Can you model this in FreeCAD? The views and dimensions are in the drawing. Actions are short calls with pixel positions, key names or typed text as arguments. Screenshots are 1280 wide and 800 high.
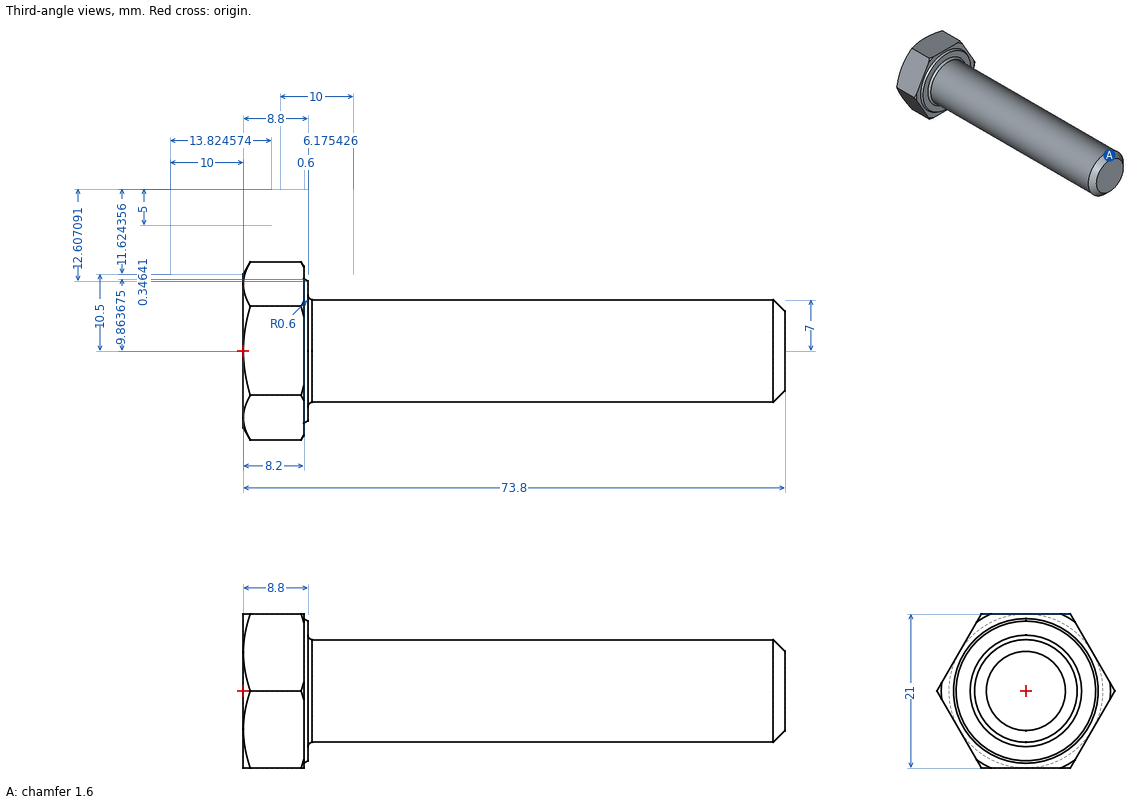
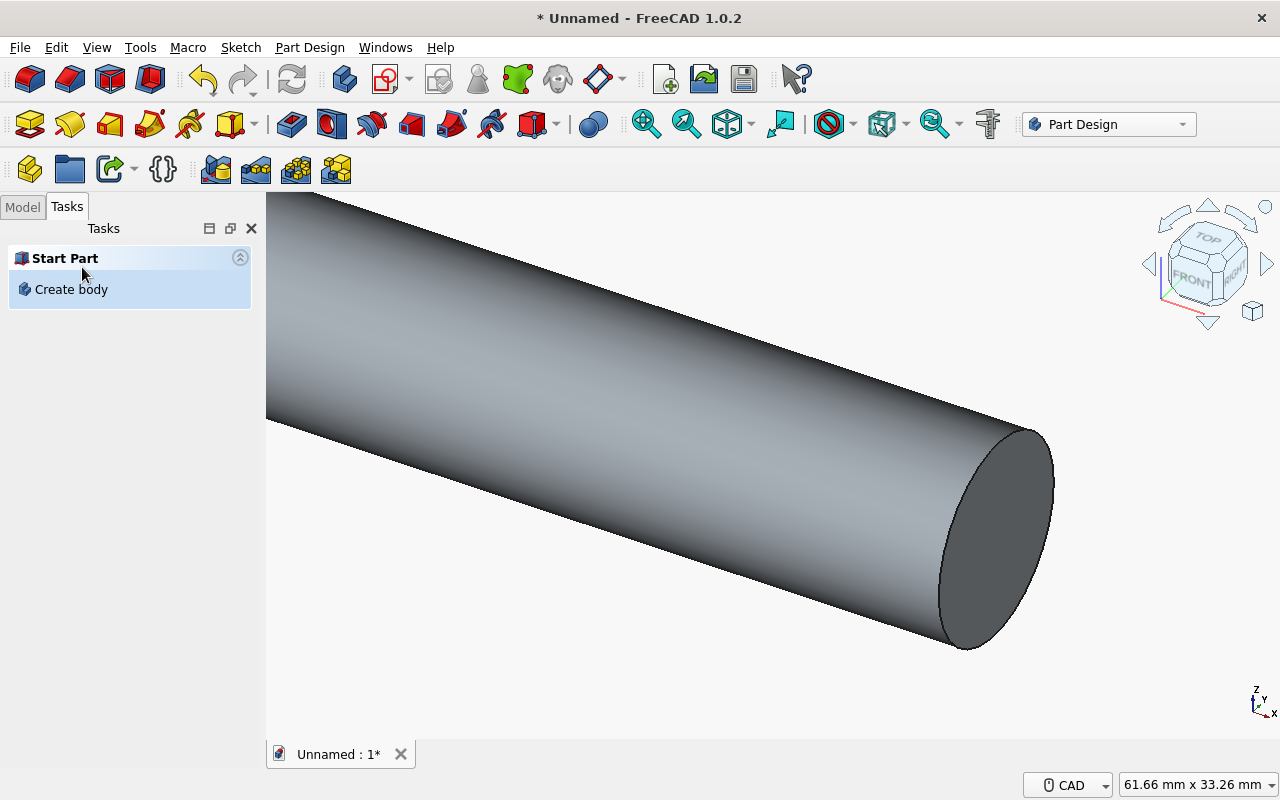
click(648, 124)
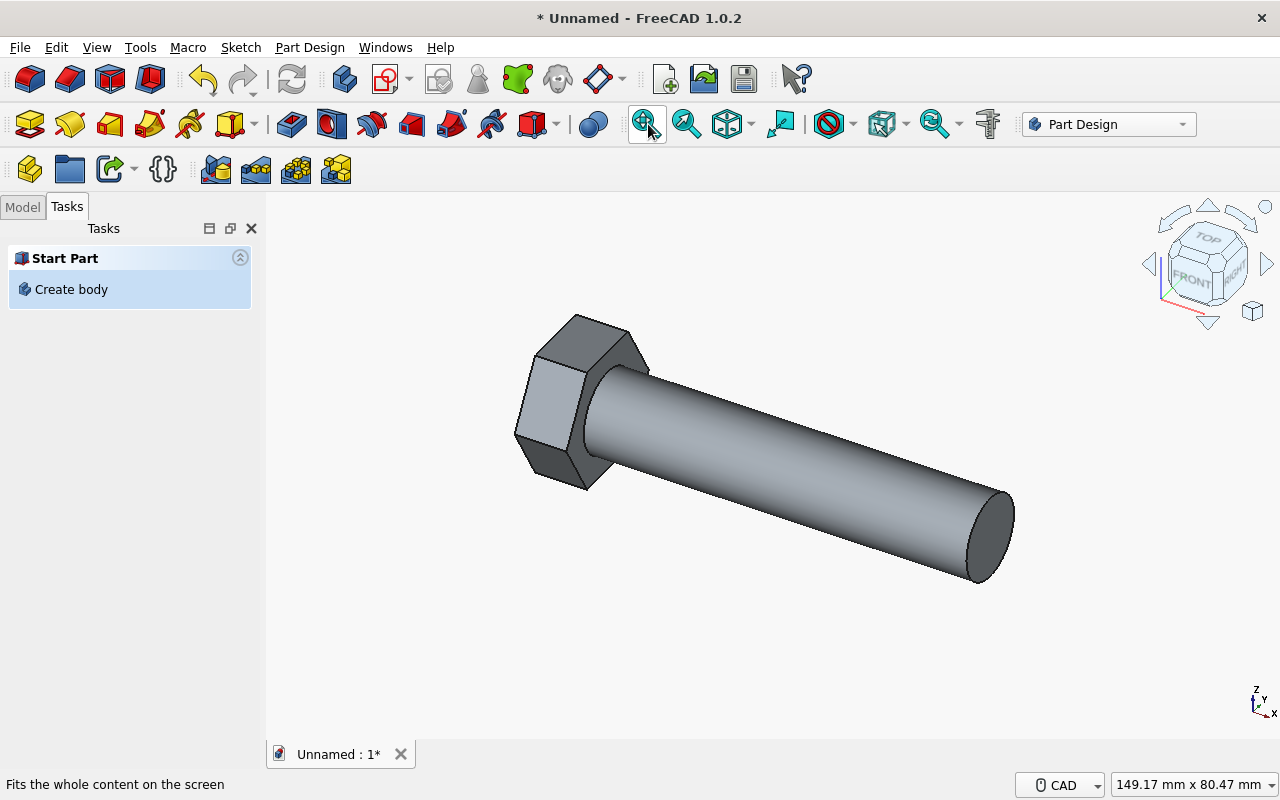
click(386, 80)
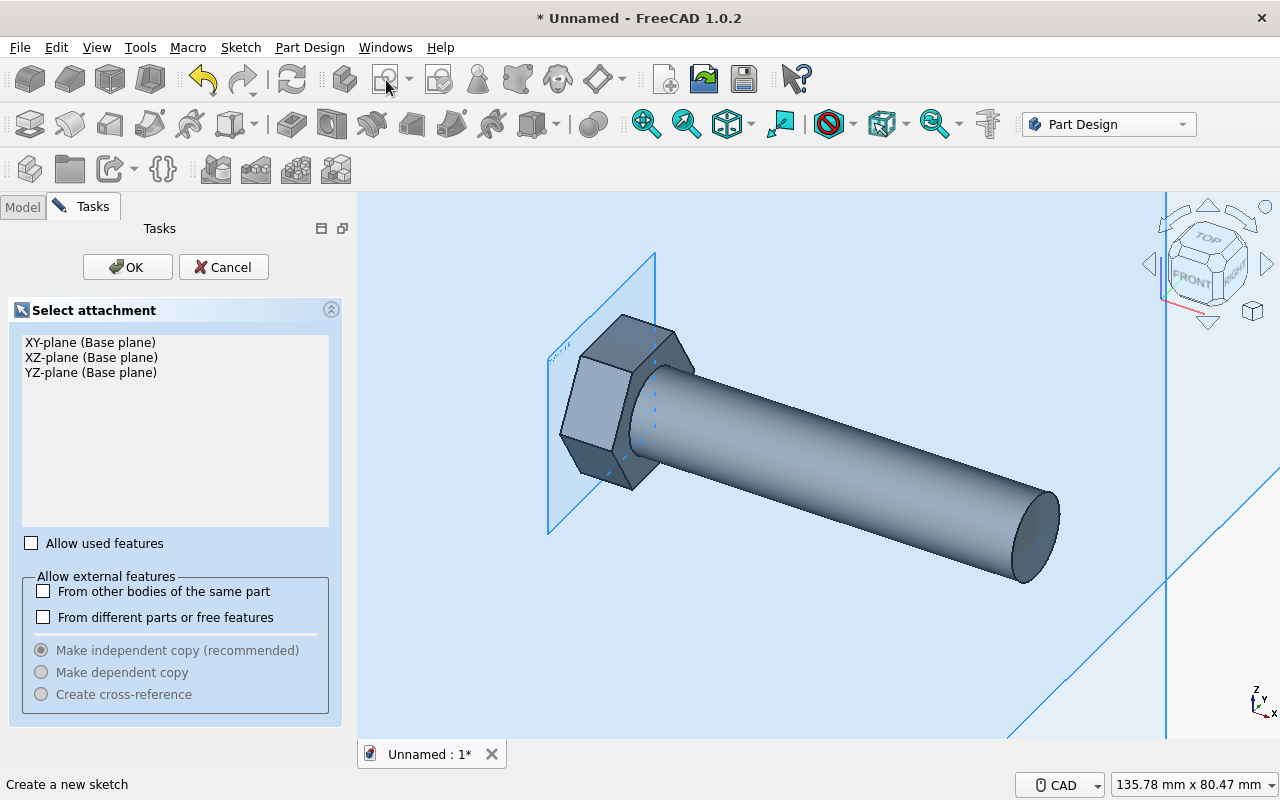
click(82, 342)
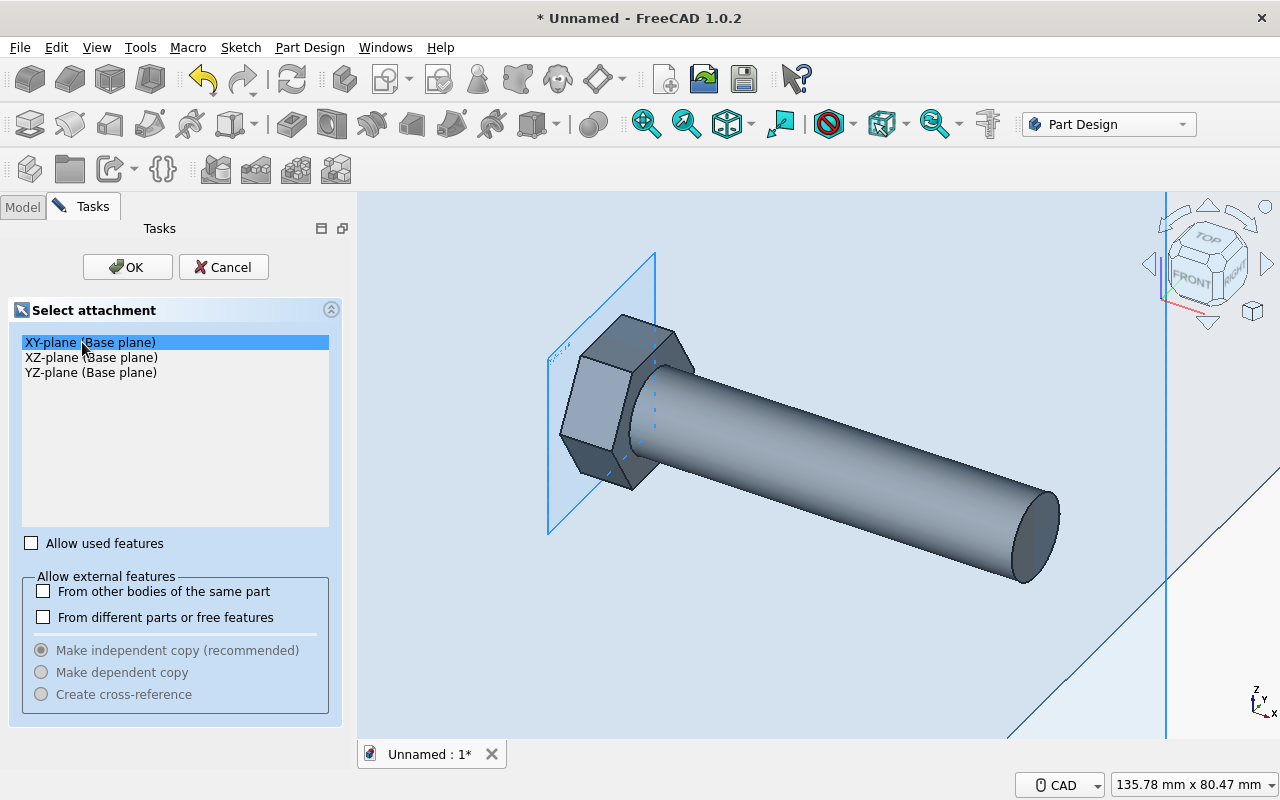
click(128, 267)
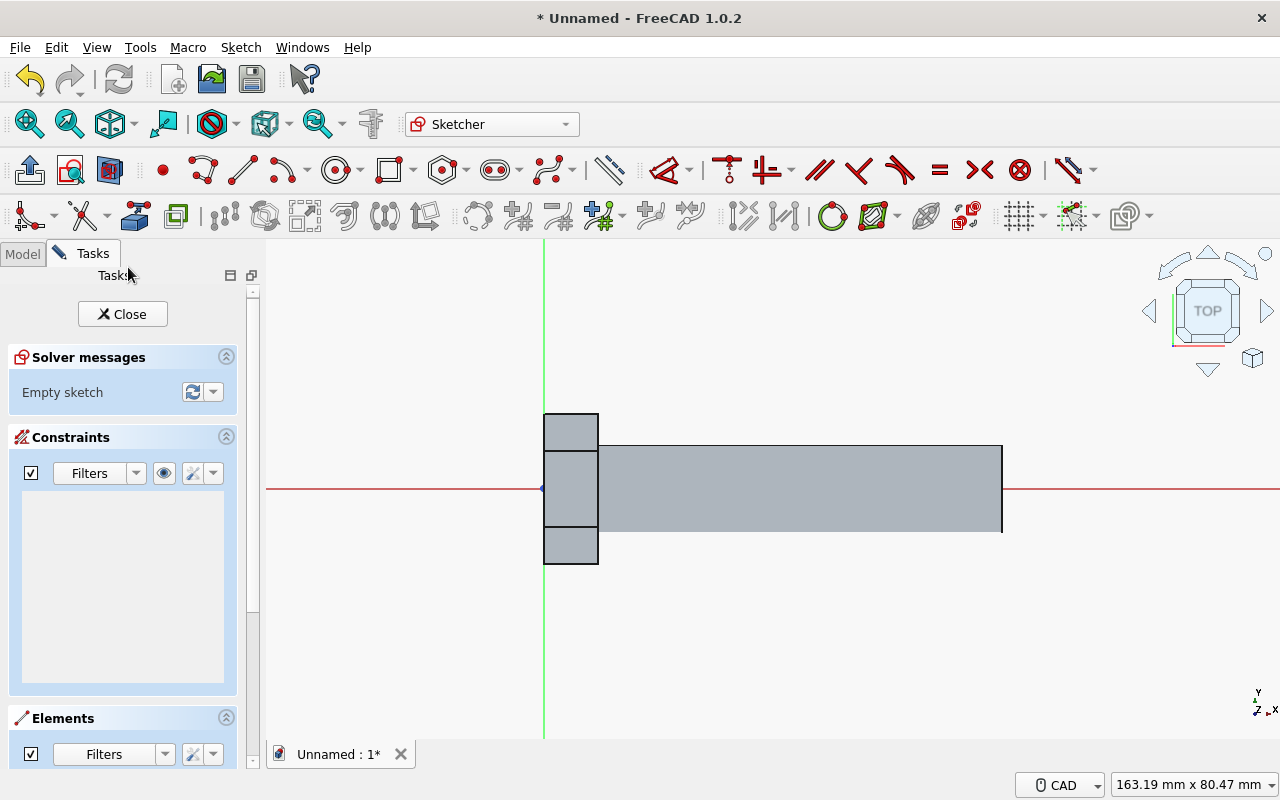
click(110, 170)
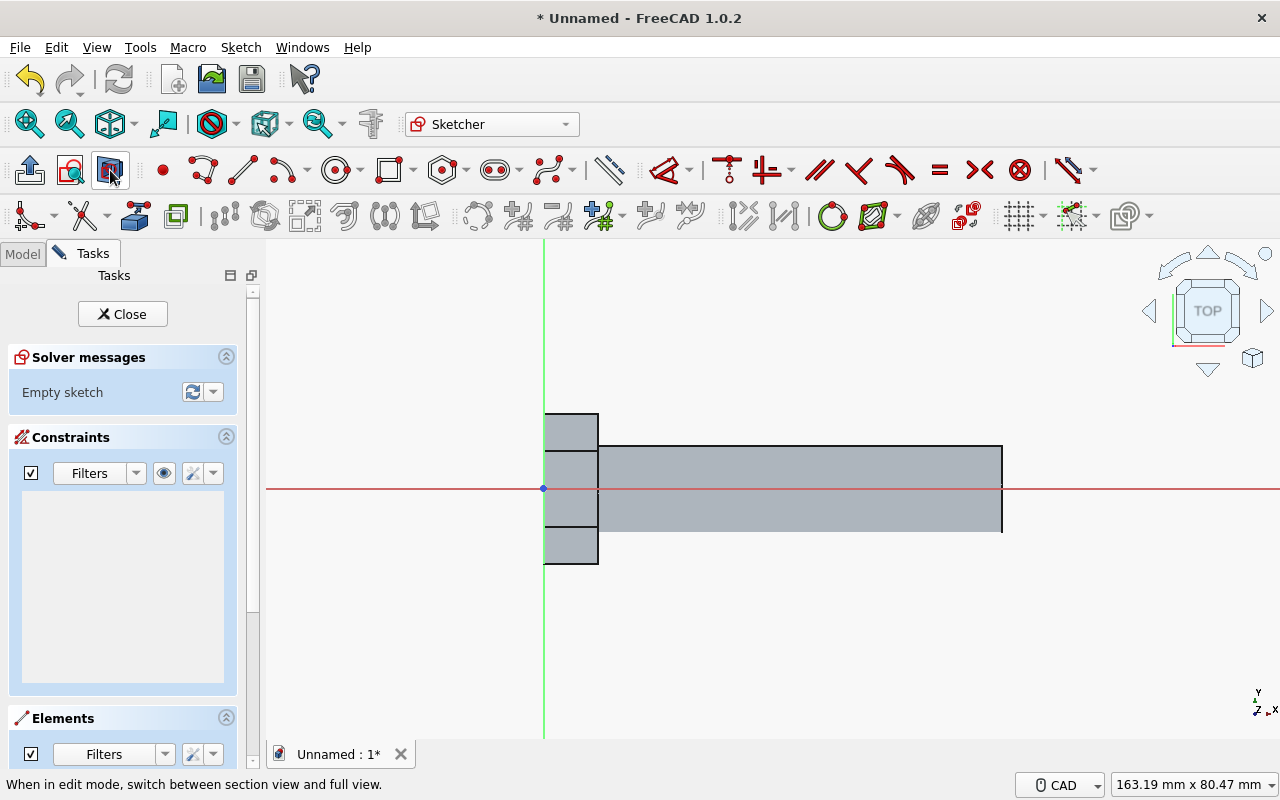
scroll(378, 364, up, 4)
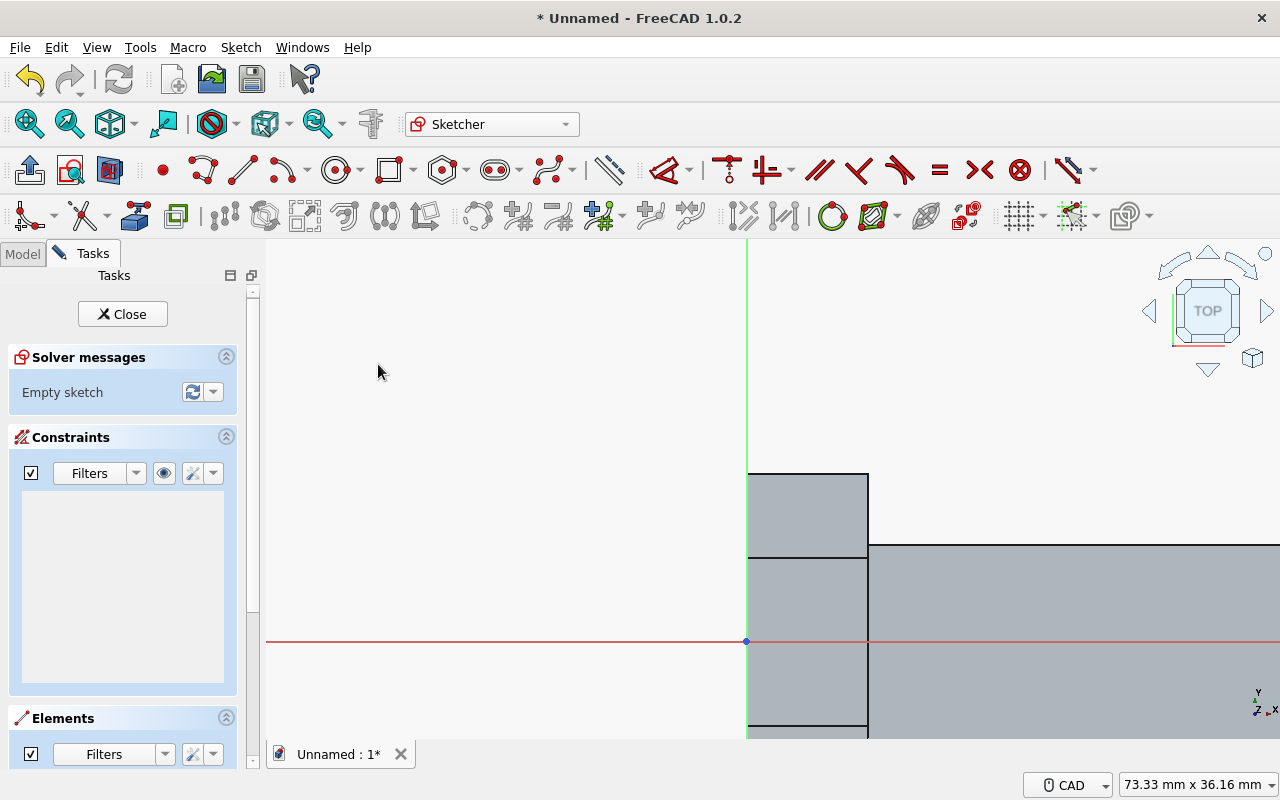
click(204, 170)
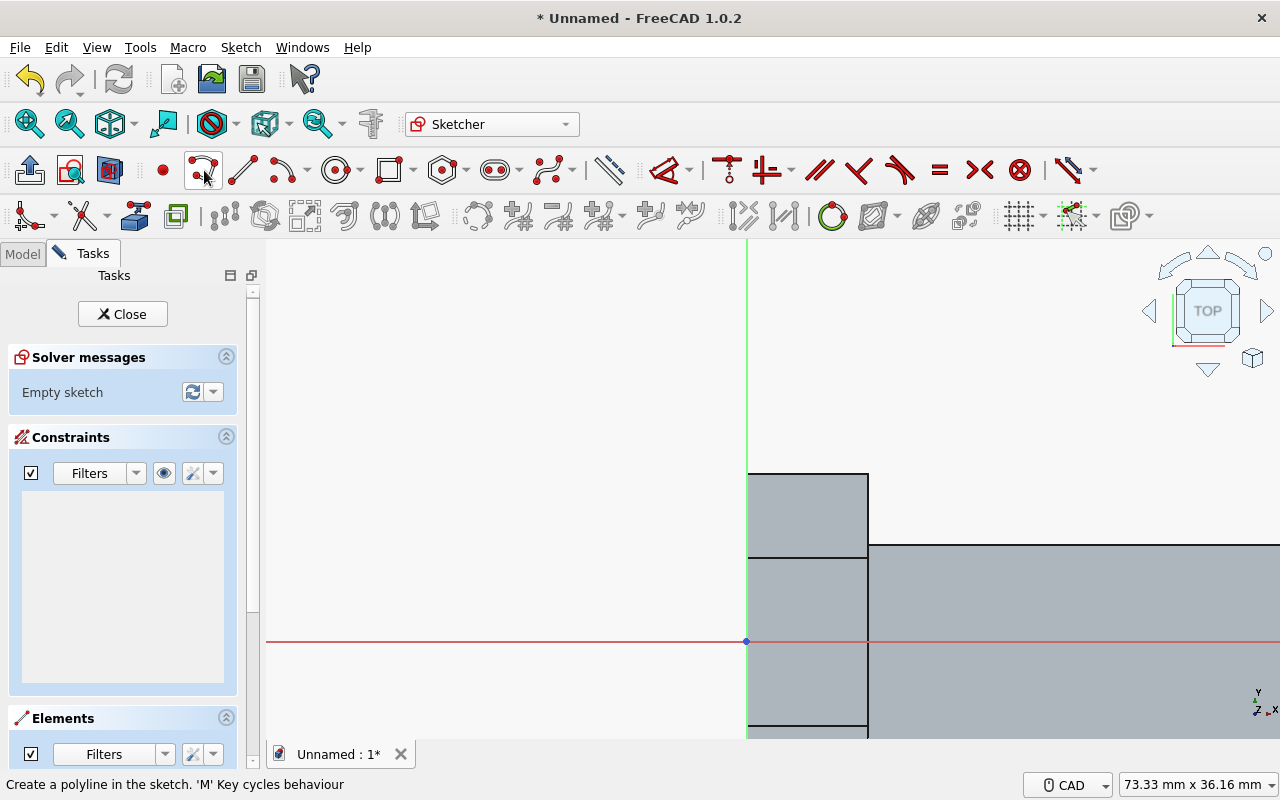
click(747, 497)
click(800, 405)
click(800, 336)
click(608, 336)
click(608, 497)
click(747, 498)
key(Escape)
key(Escape)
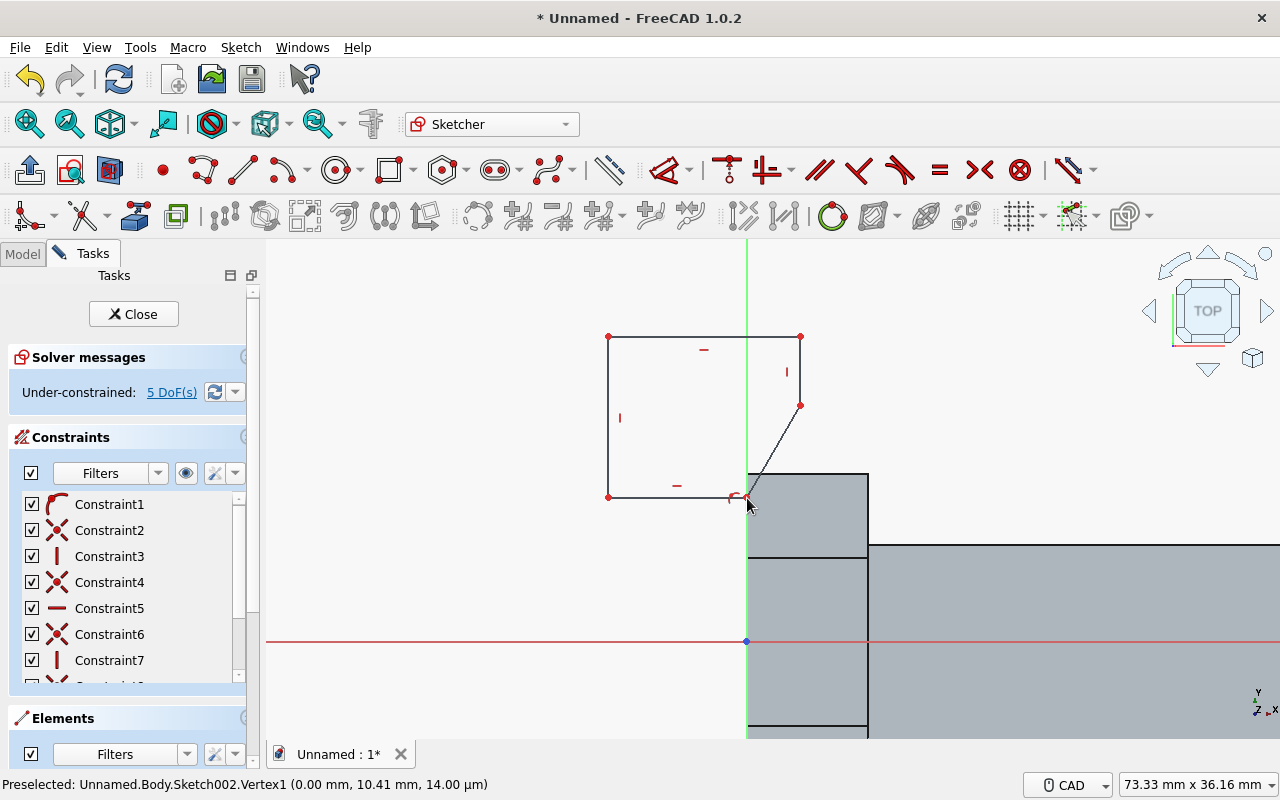
click(664, 170)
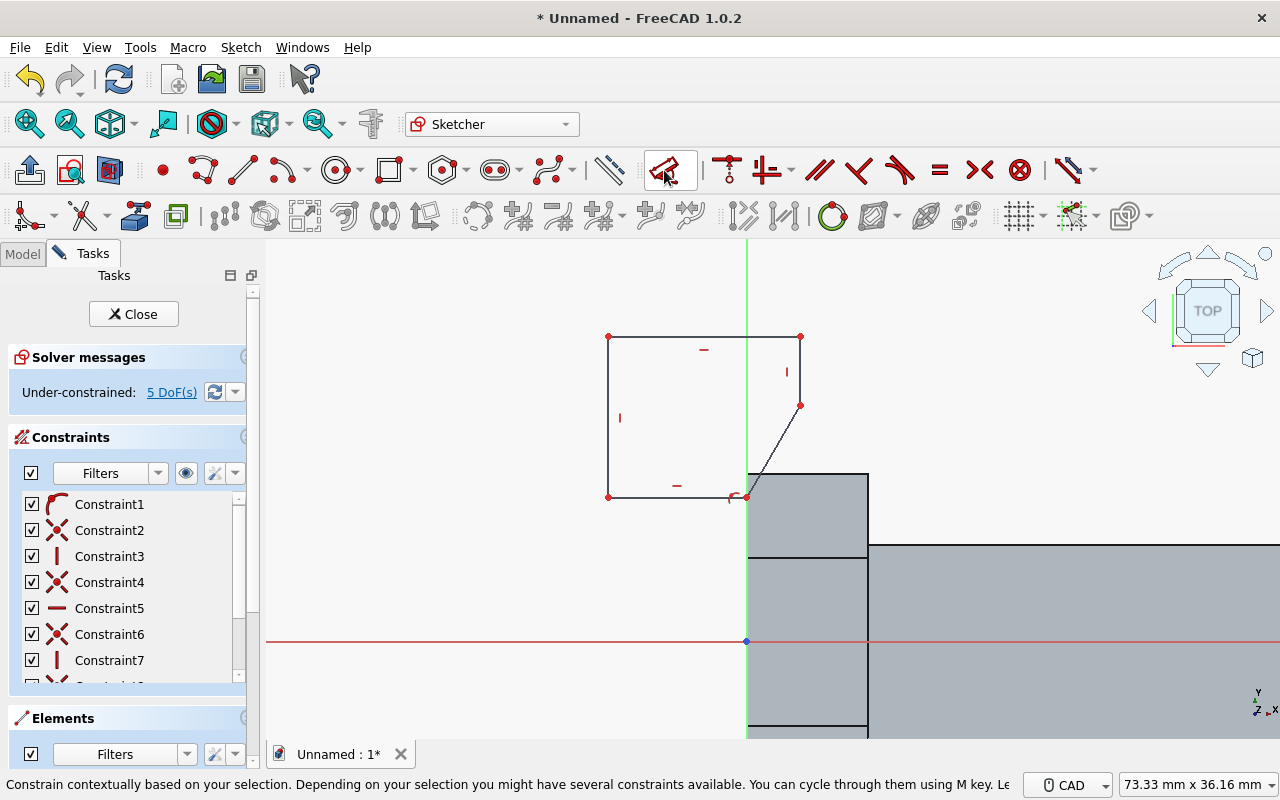
click(800, 385)
click(834, 371)